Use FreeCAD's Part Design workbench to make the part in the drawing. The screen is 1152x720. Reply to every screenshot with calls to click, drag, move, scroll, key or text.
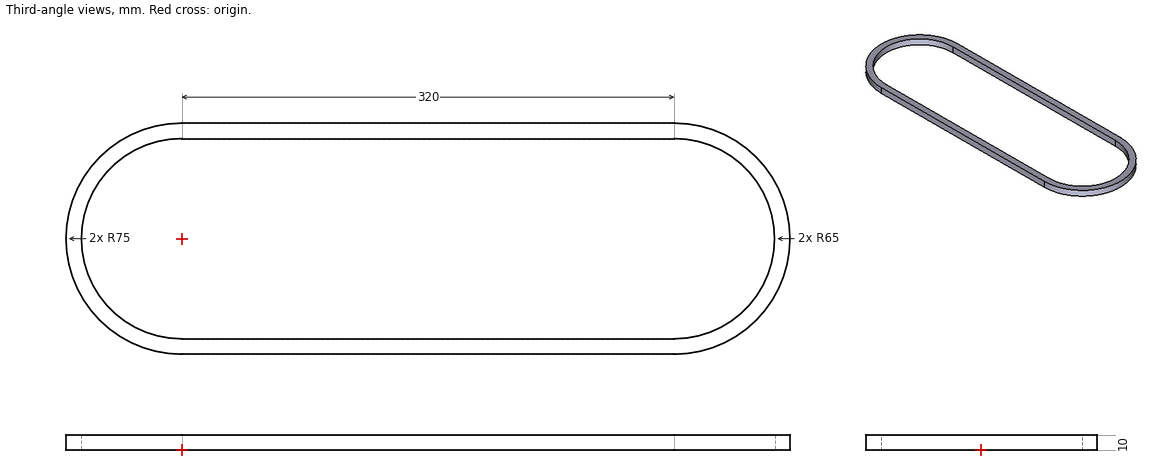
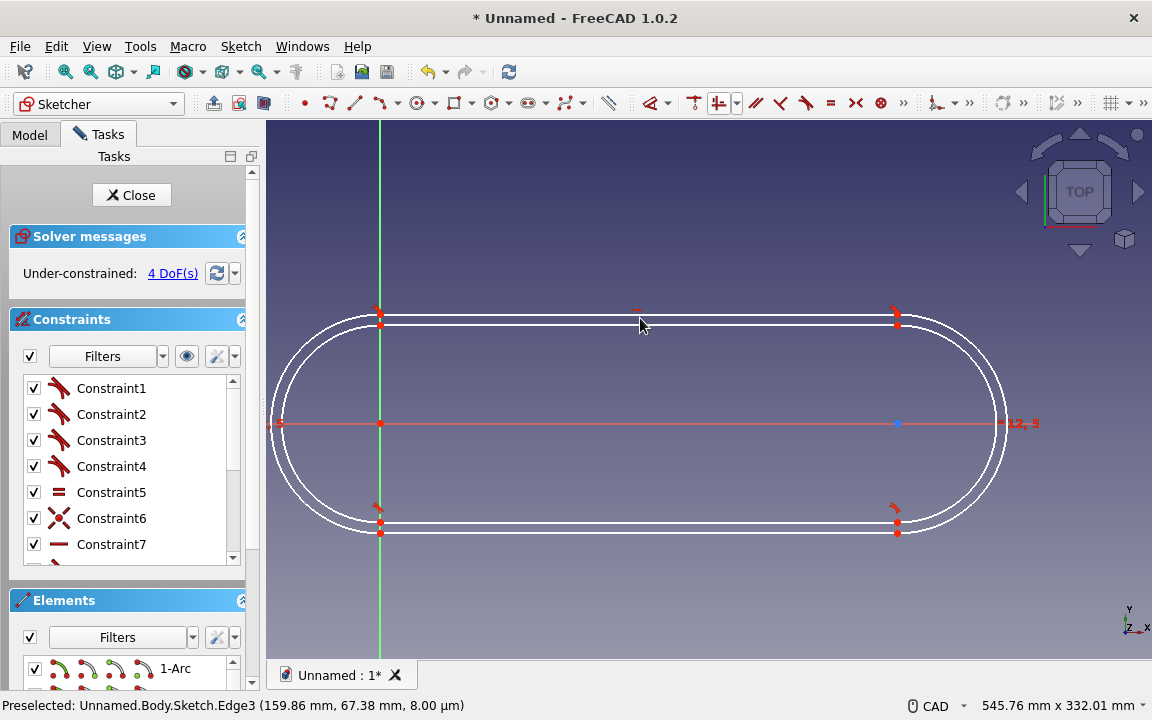
scroll(316, 336, up, 2)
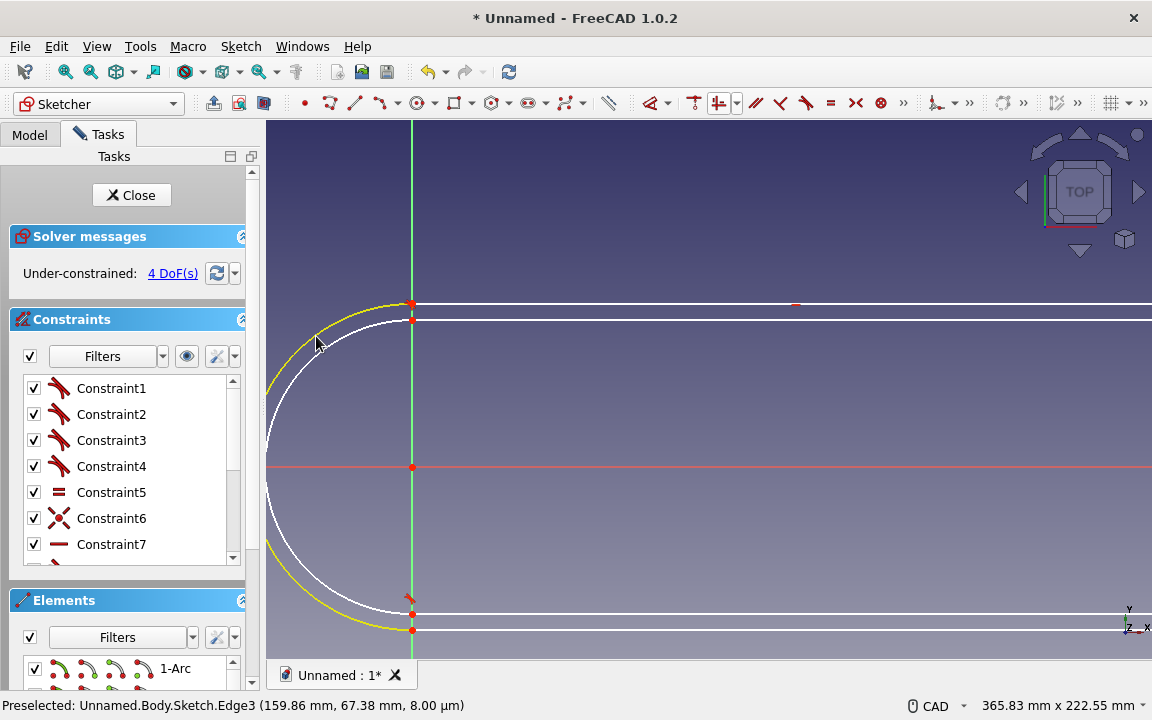
click(316, 335)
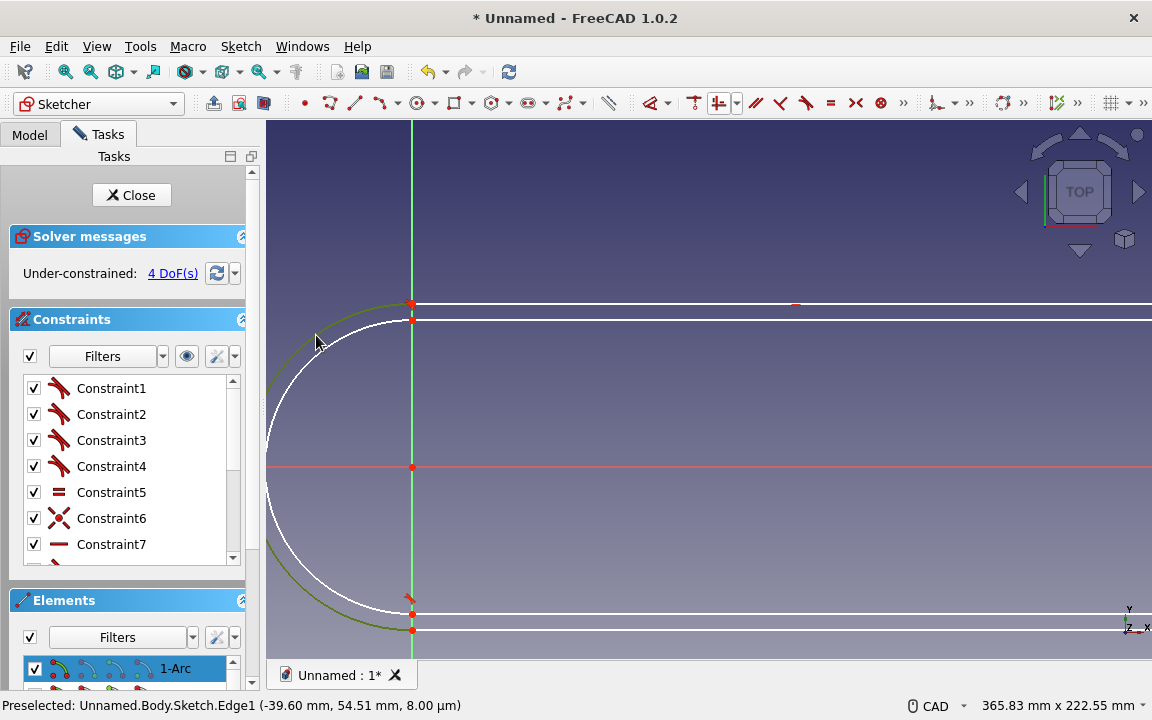
click(668, 104)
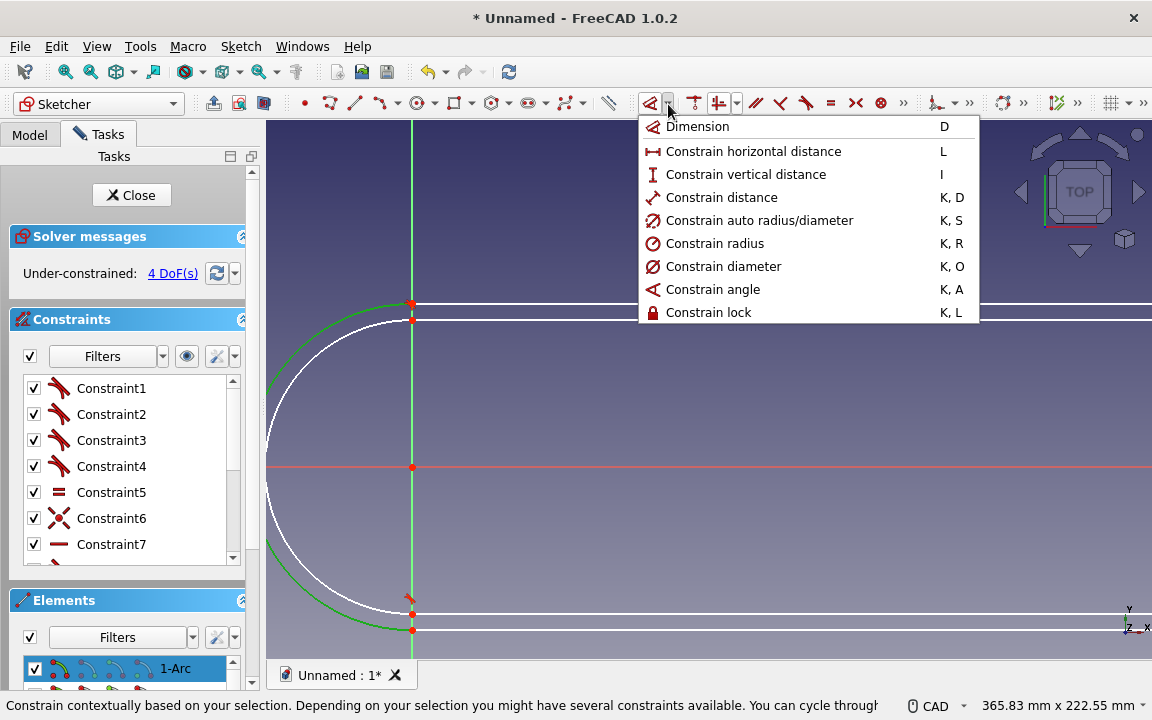
click(809, 244)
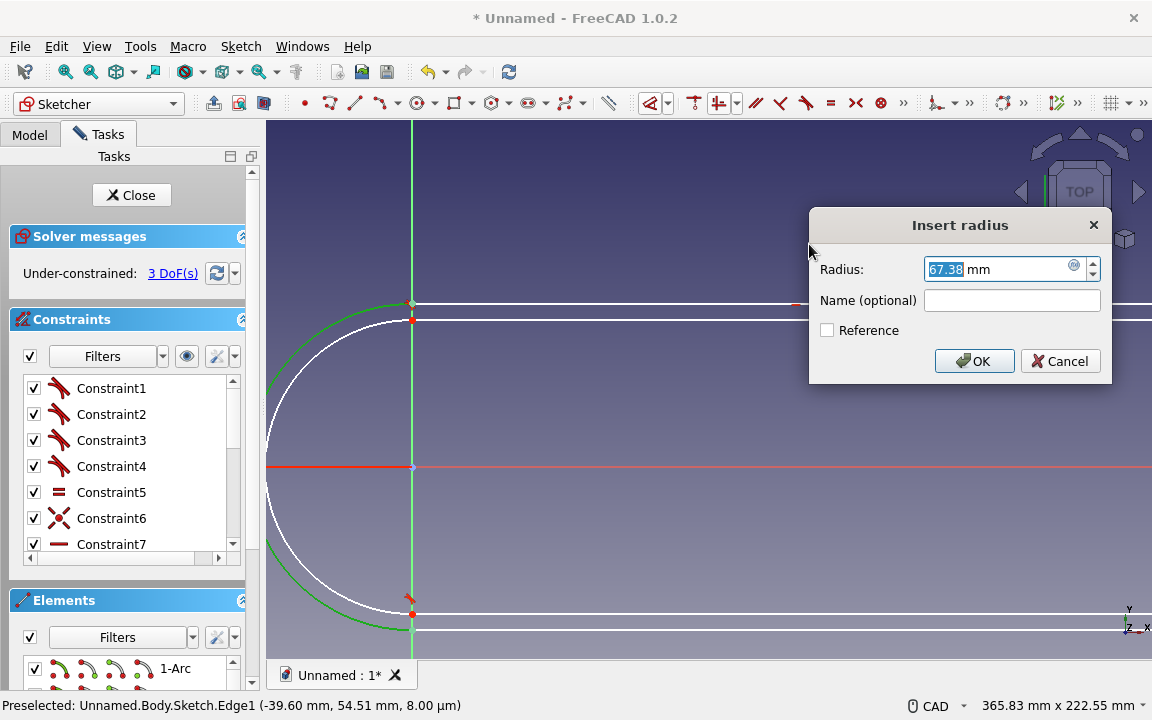
text(65)
key(Return)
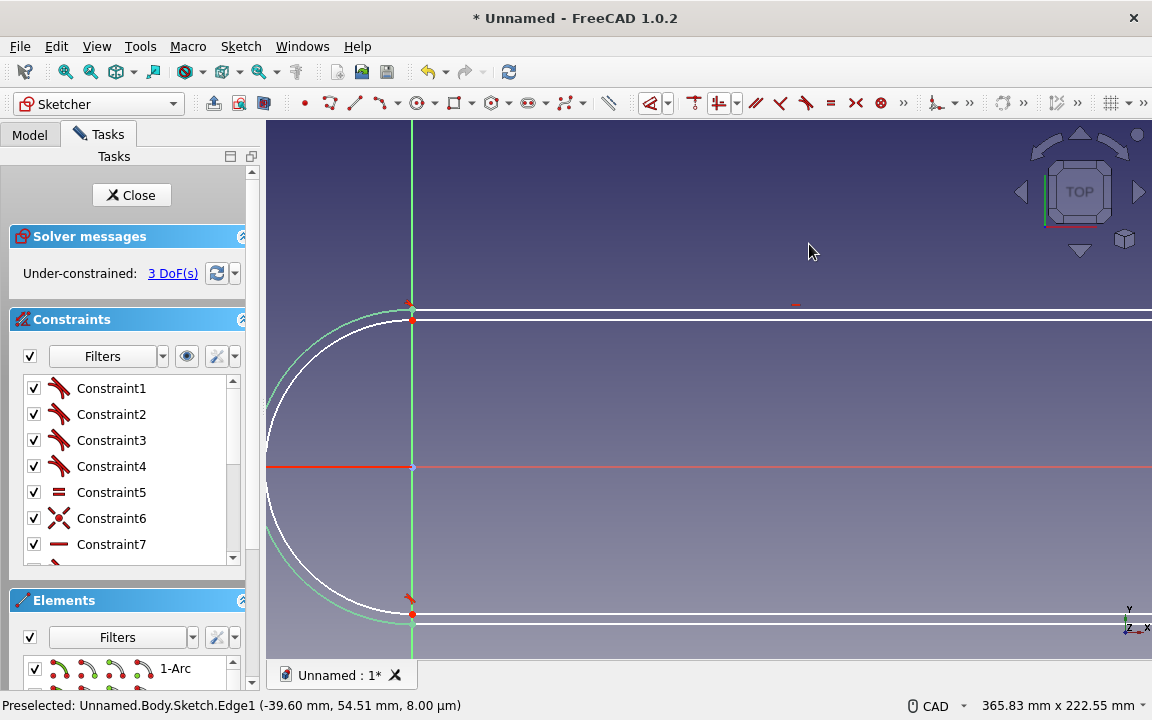
scroll(326, 348, up, 2)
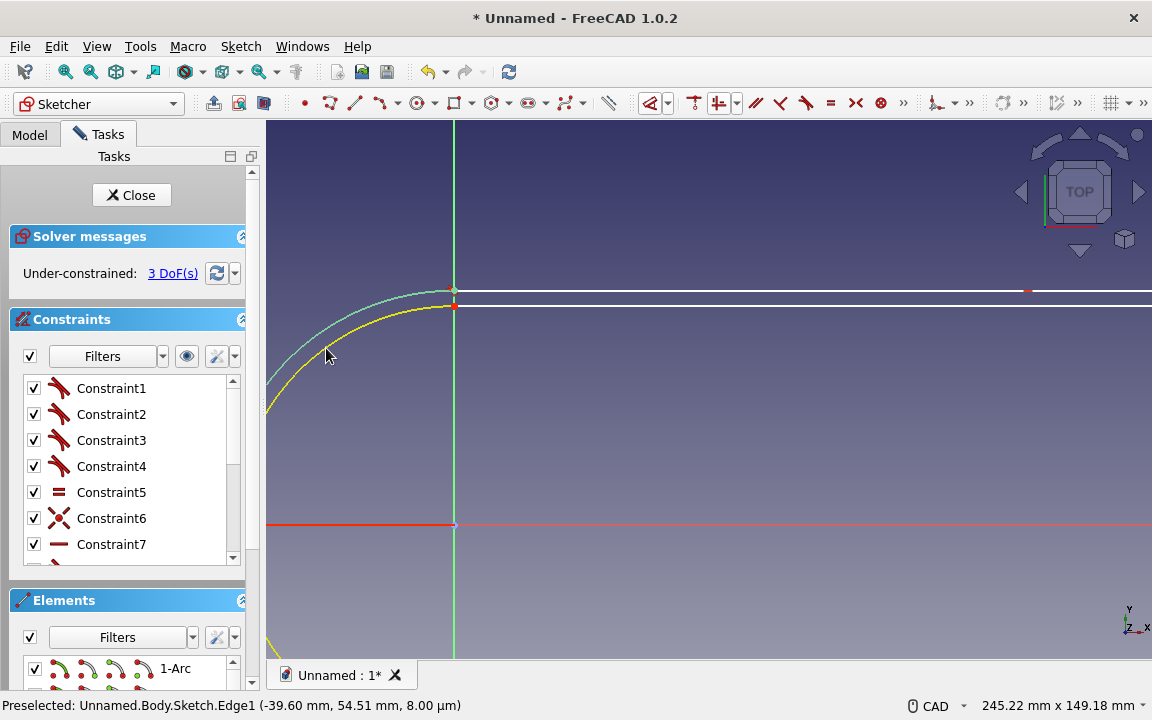
click(326, 348)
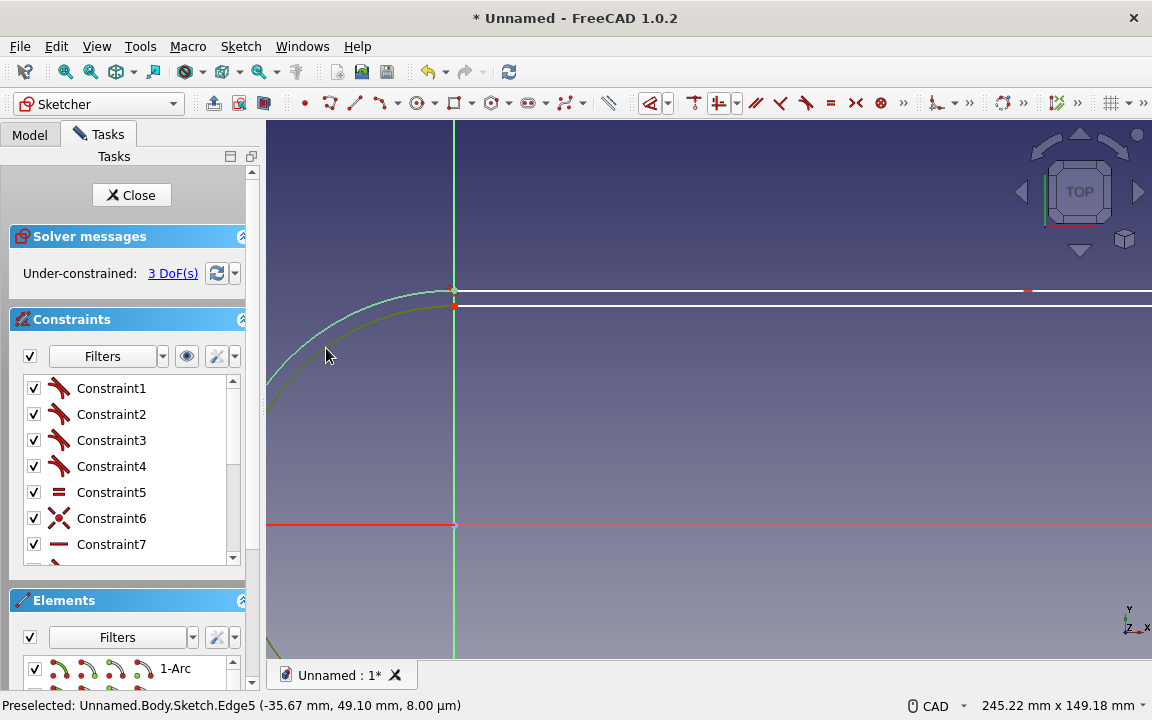
key(k)
key(r)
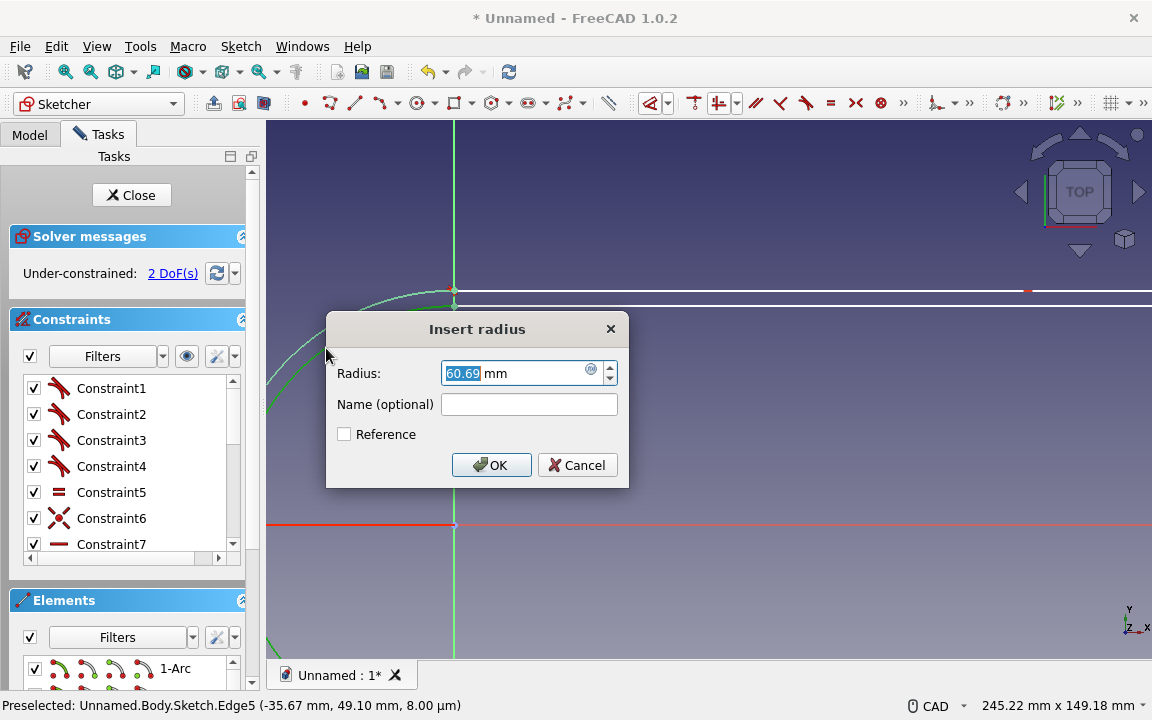
text(75)
key(Return)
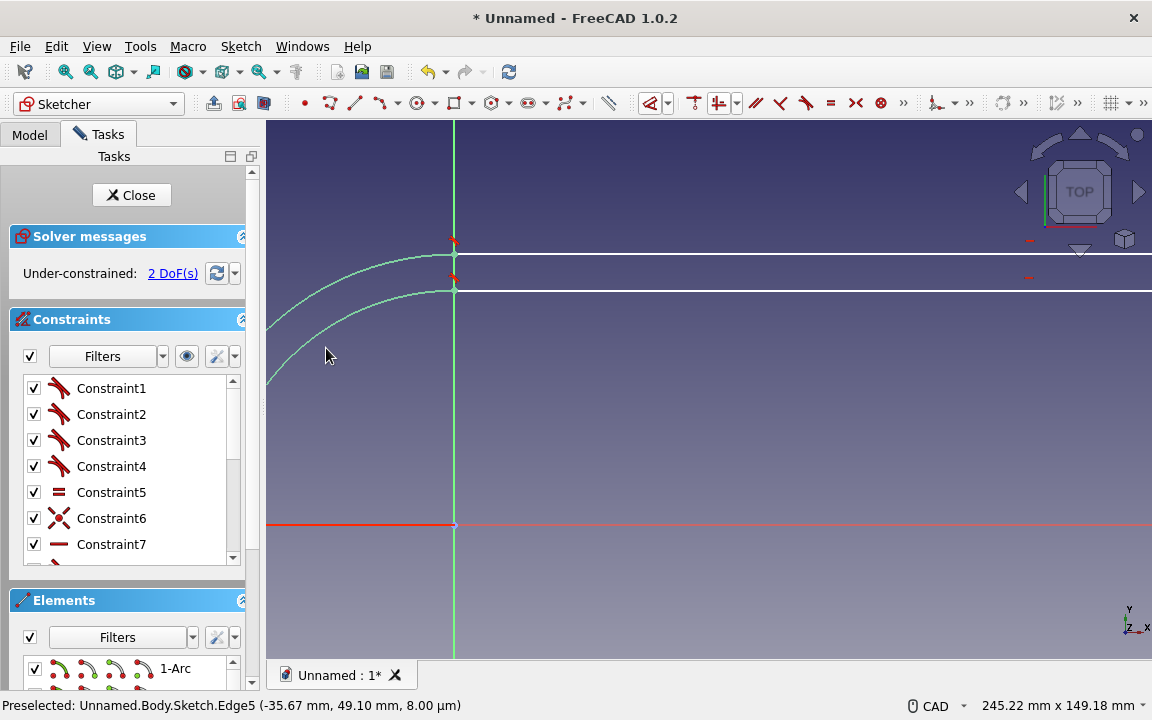
click(800, 291)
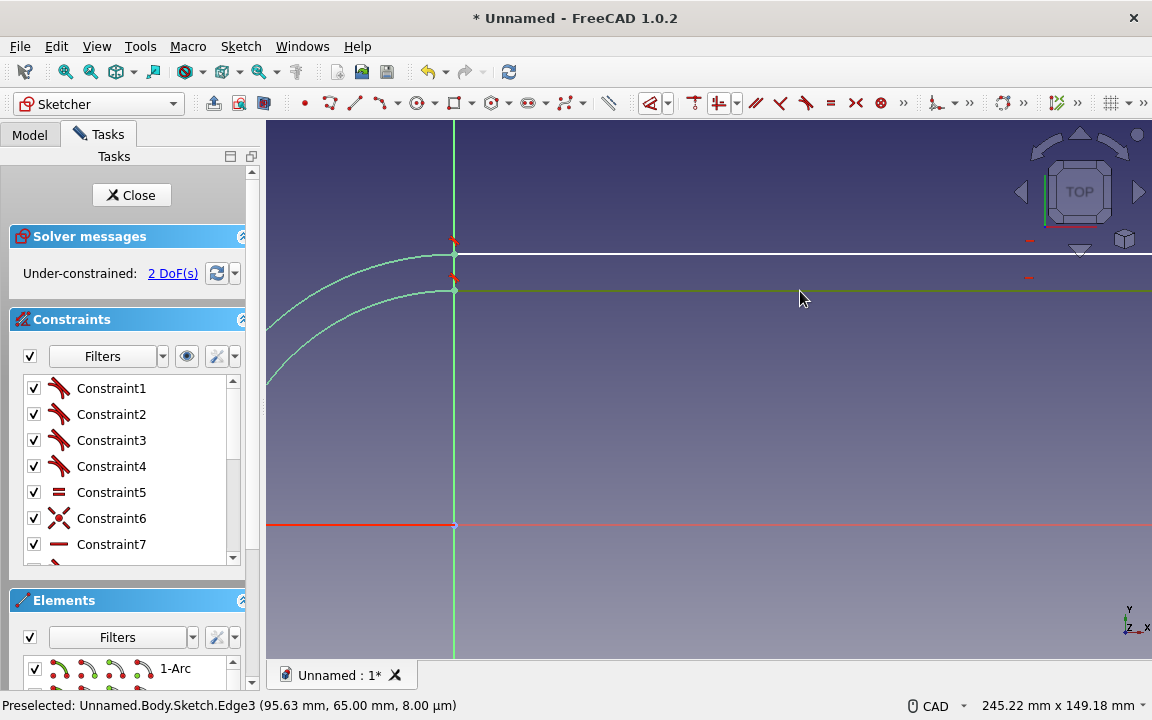
click(668, 104)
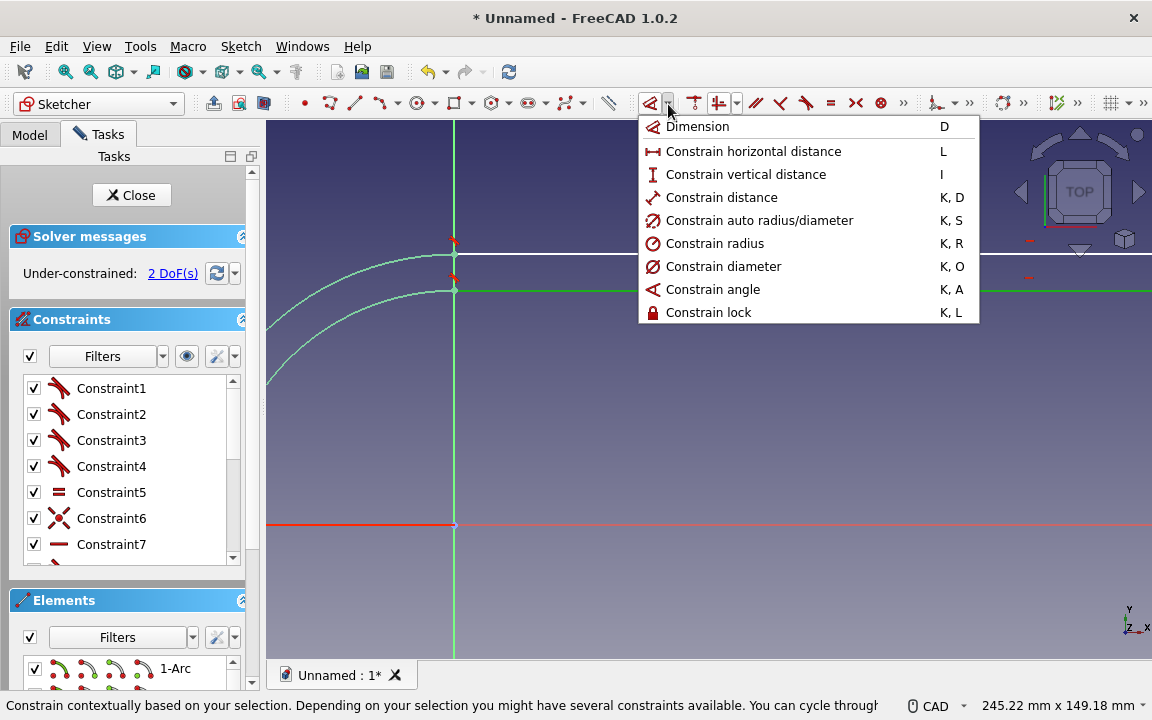
click(809, 152)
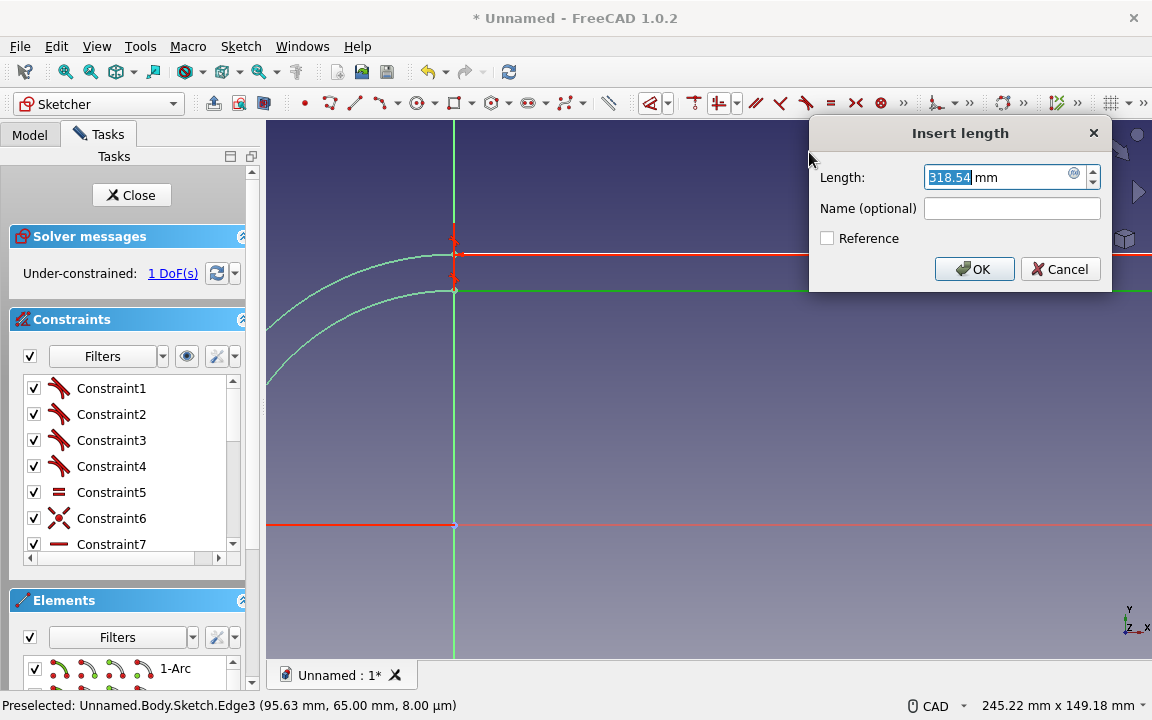
text(320)
key(Return)